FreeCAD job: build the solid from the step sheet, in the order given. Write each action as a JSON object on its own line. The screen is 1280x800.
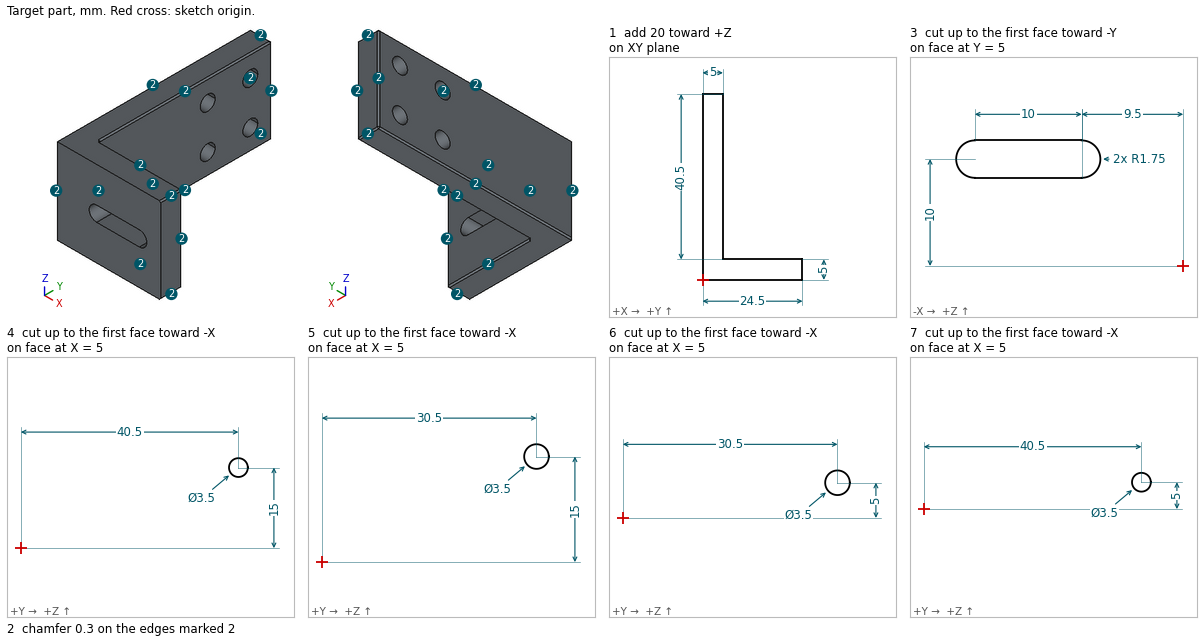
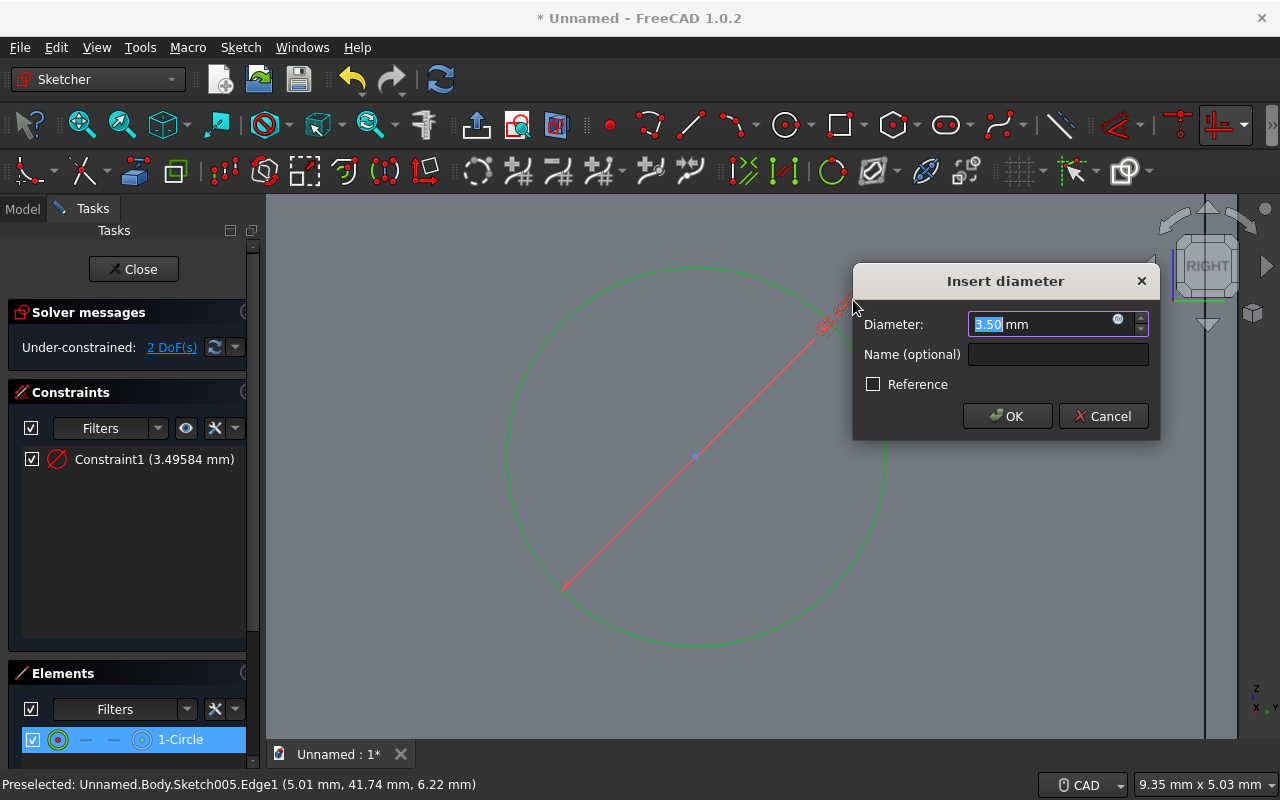
{"action": "type", "text": "3.5"}
{"action": "key", "text": "Return"}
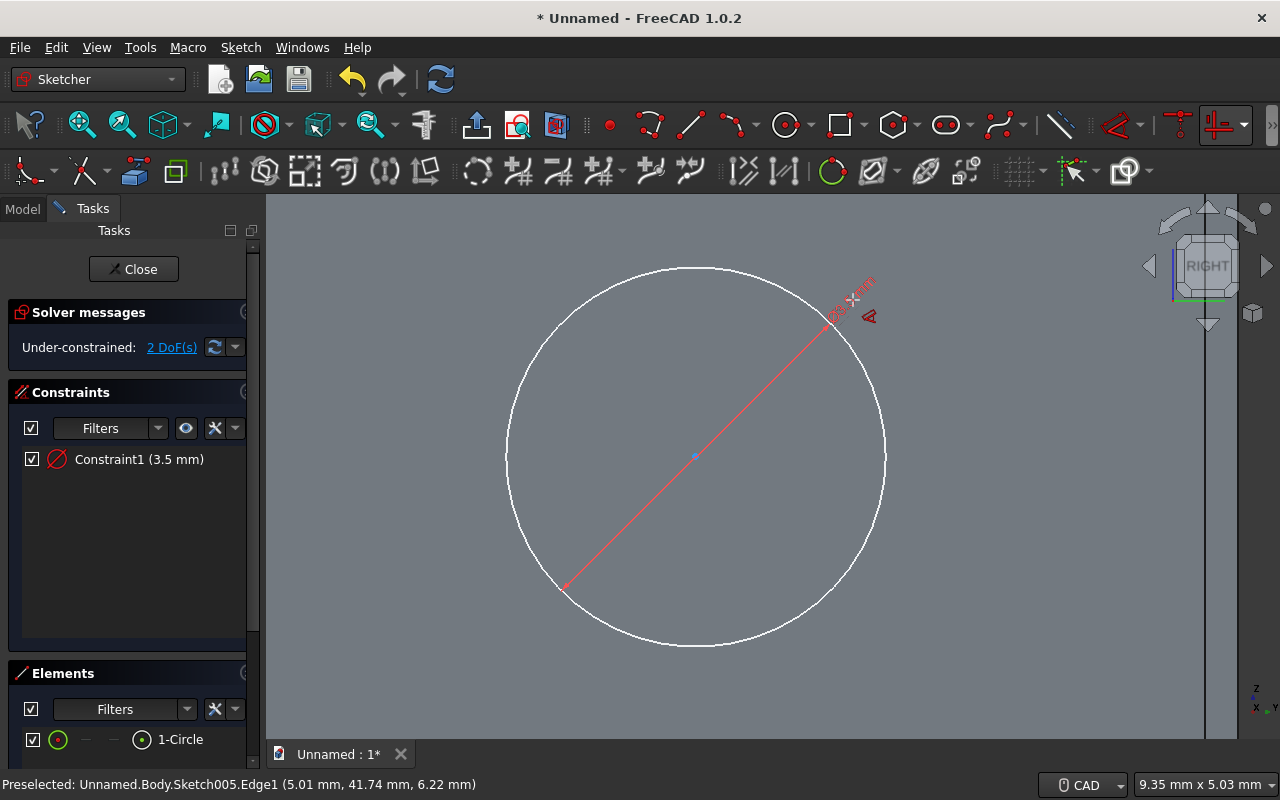
{"action": "left_click", "coordinate": [696, 457]}
{"action": "left_click", "coordinate": [730, 584]}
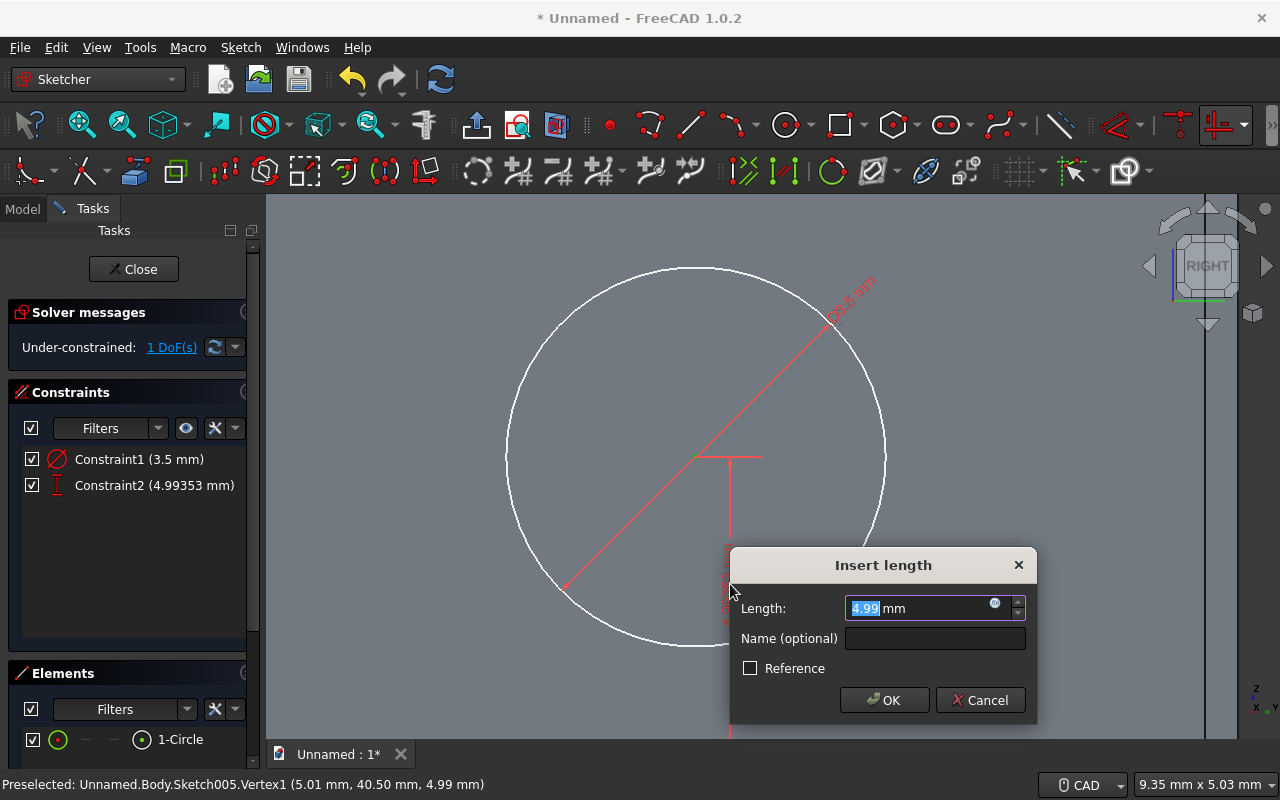
{"action": "type", "text": "5"}
{"action": "key", "text": "Return"}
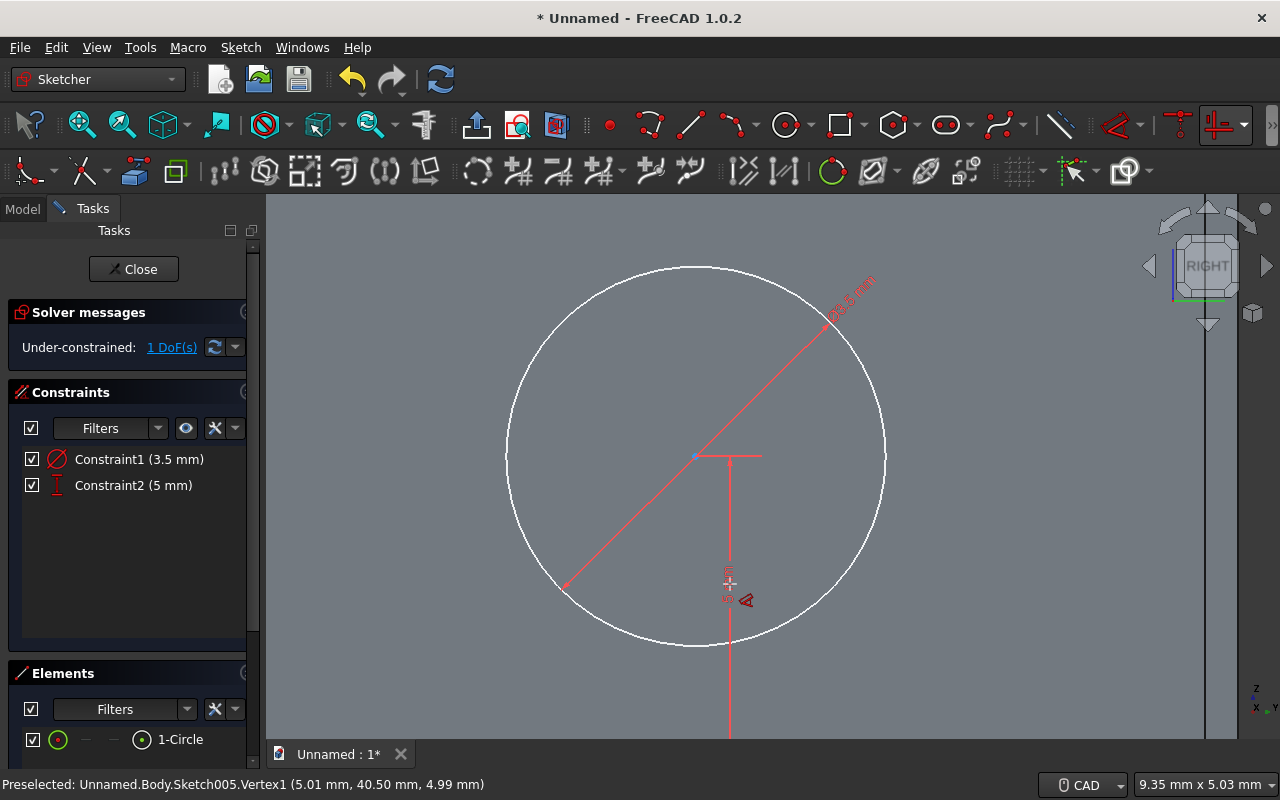
{"action": "left_click", "coordinate": [696, 456]}
{"action": "left_click", "coordinate": [495, 422]}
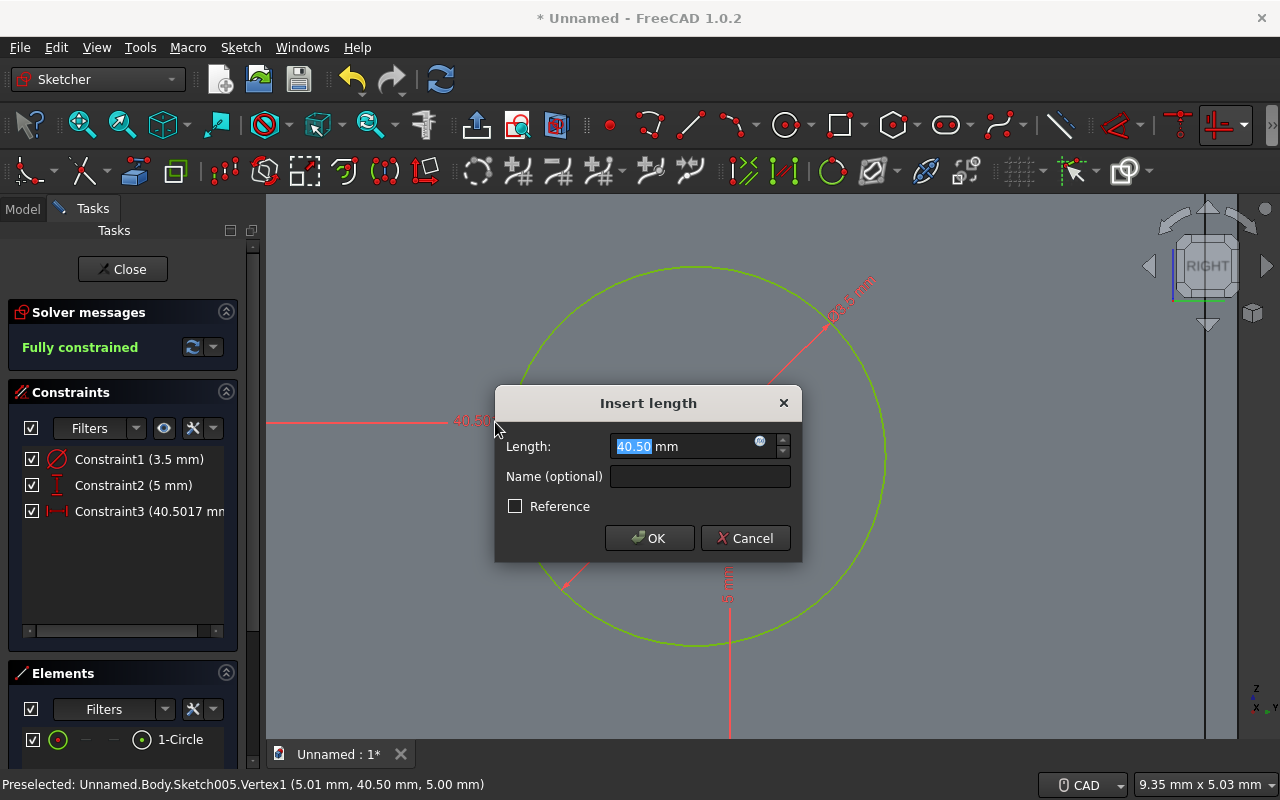
{"action": "type", "text": "40.5"}
{"action": "key", "text": "Return"}
{"action": "key", "text": "Escape"}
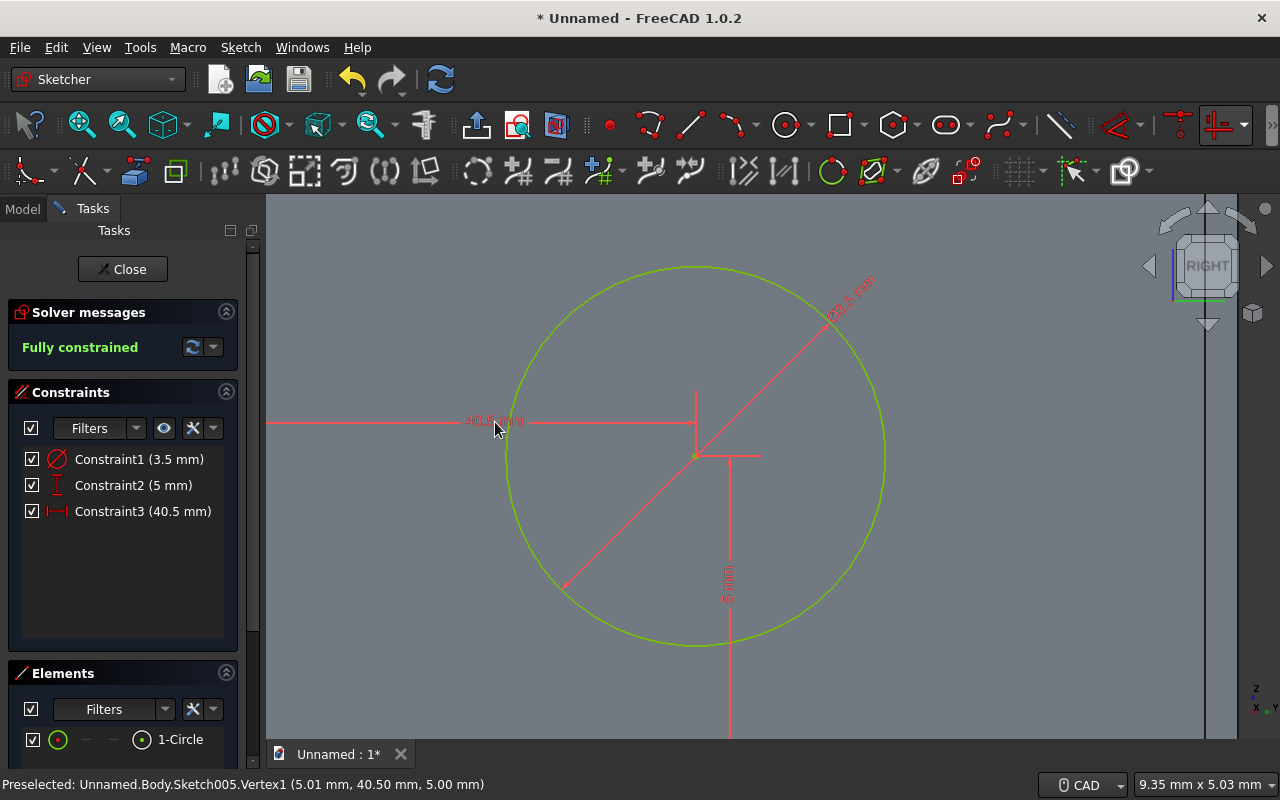
{"action": "left_click", "coordinate": [123, 269]}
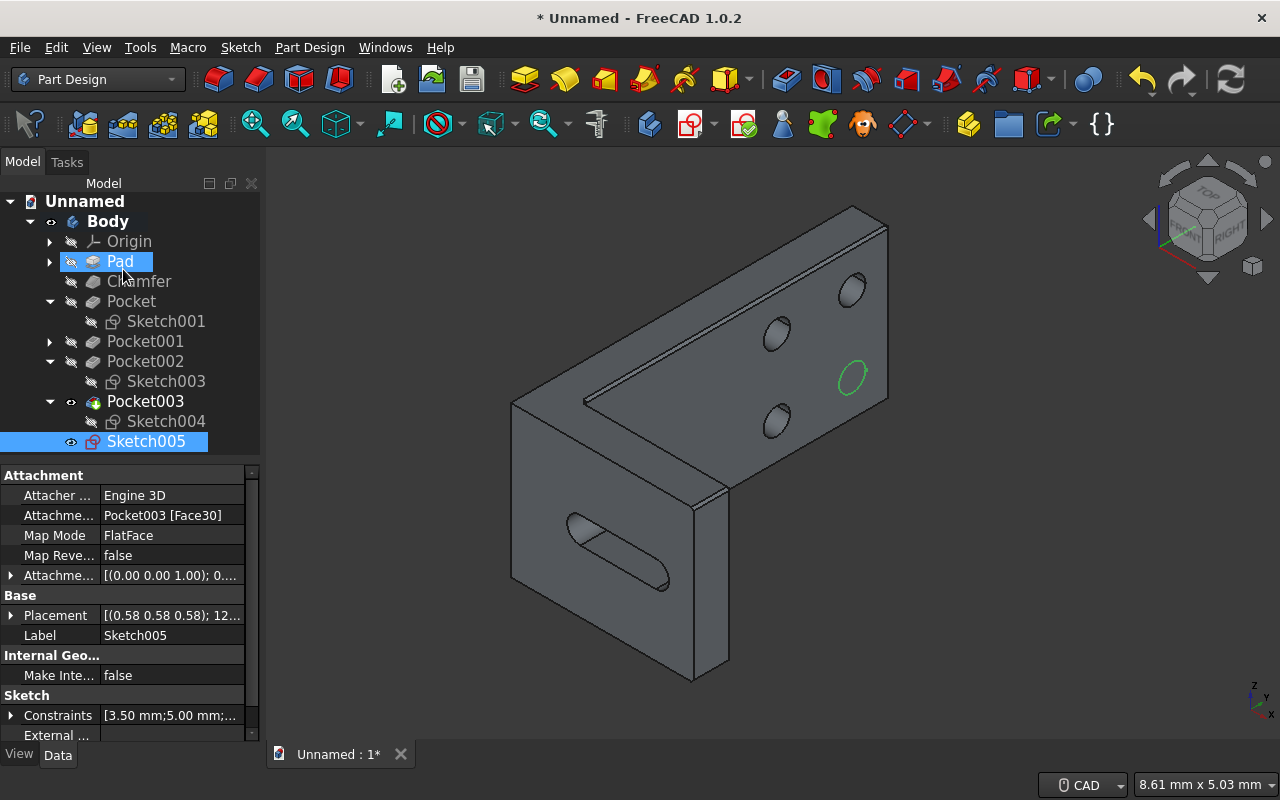
{"action": "left_click", "coordinate": [788, 80]}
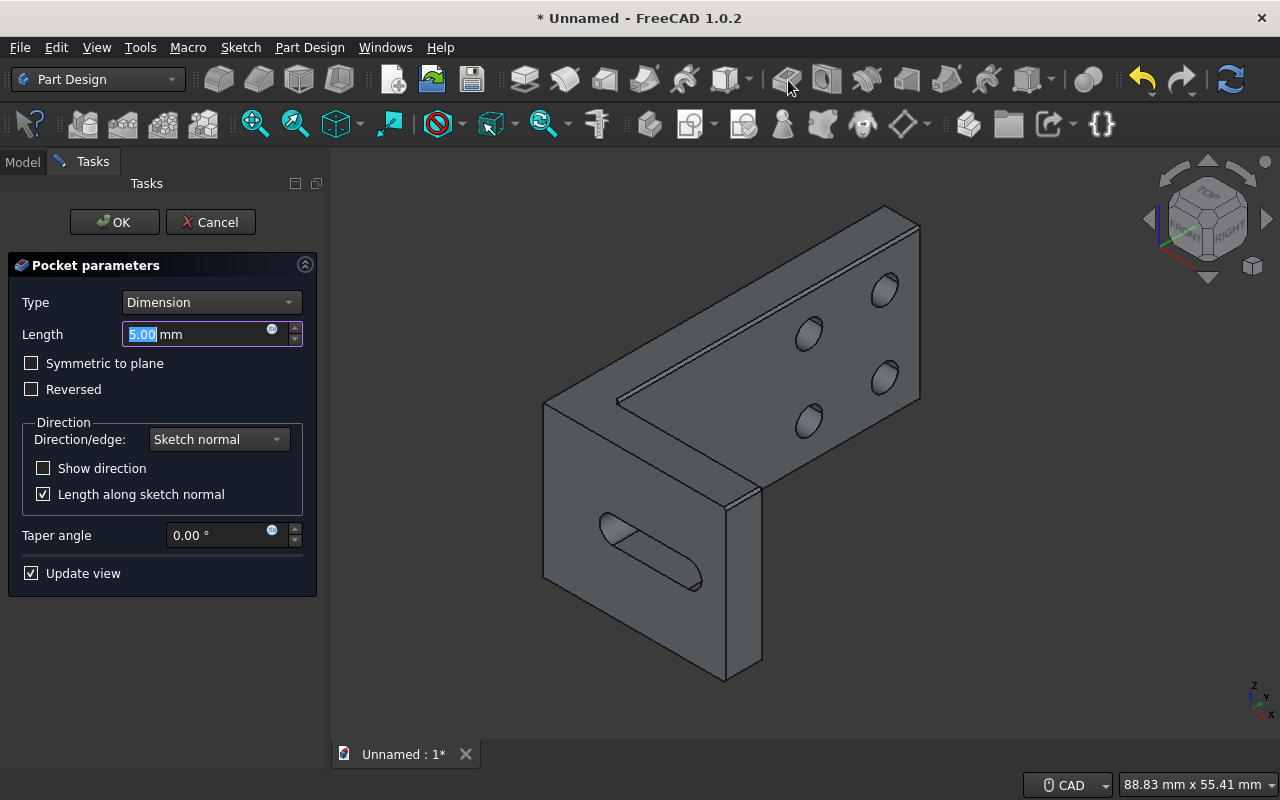
{"action": "left_click", "coordinate": [212, 302]}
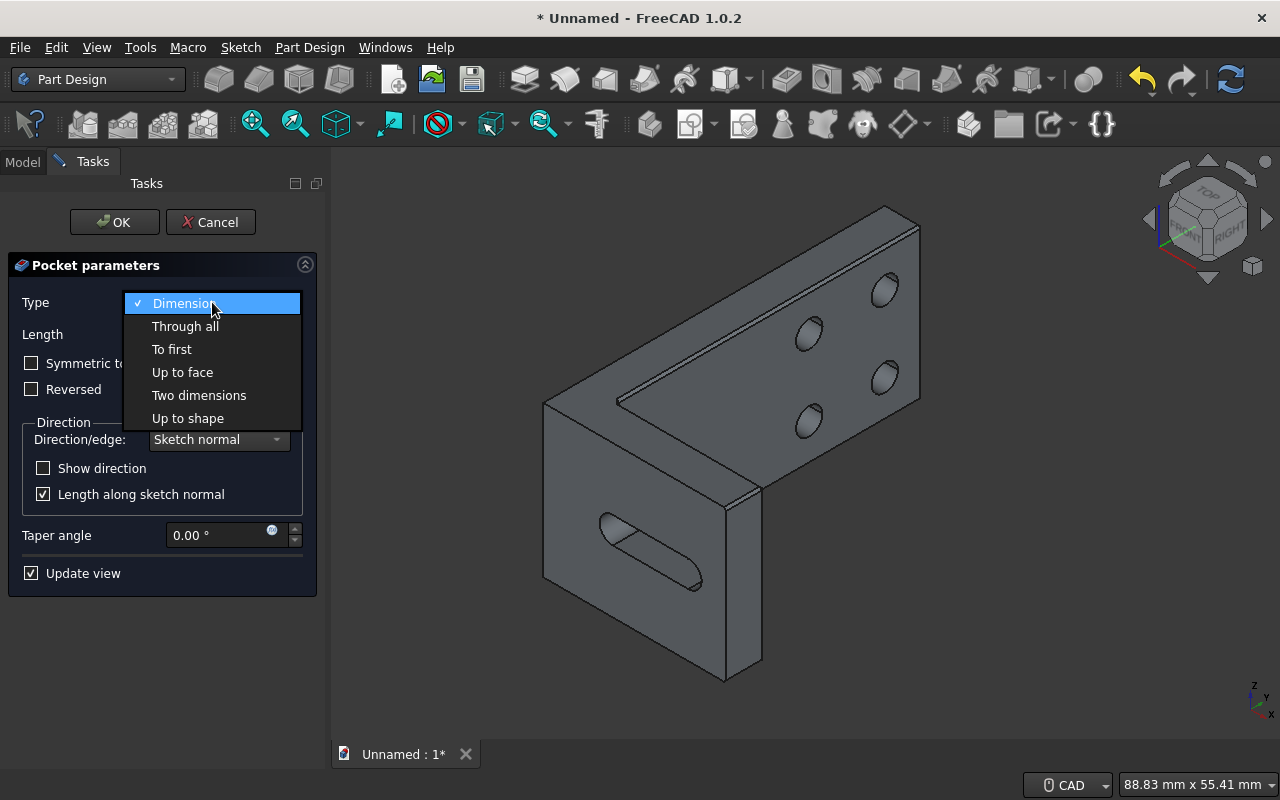
{"action": "left_click", "coordinate": [212, 350]}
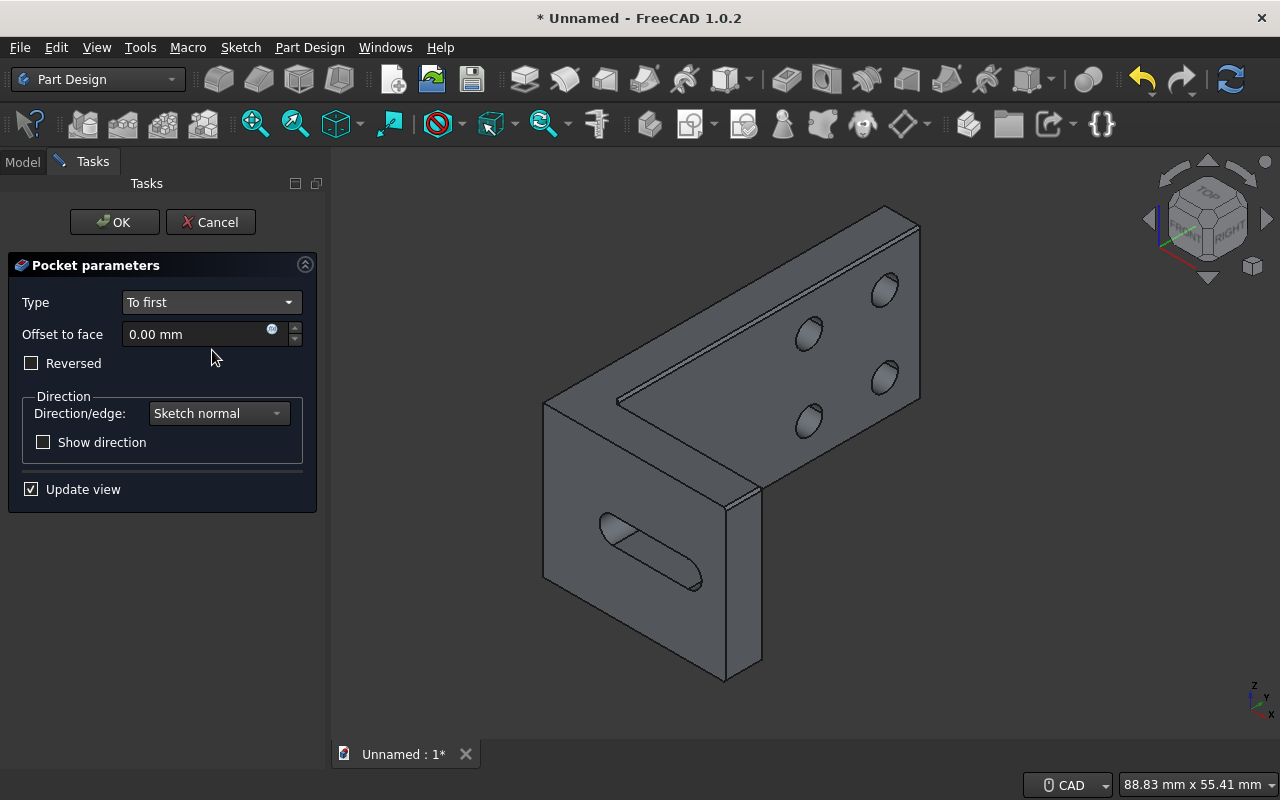
{"action": "left_click", "coordinate": [115, 222]}